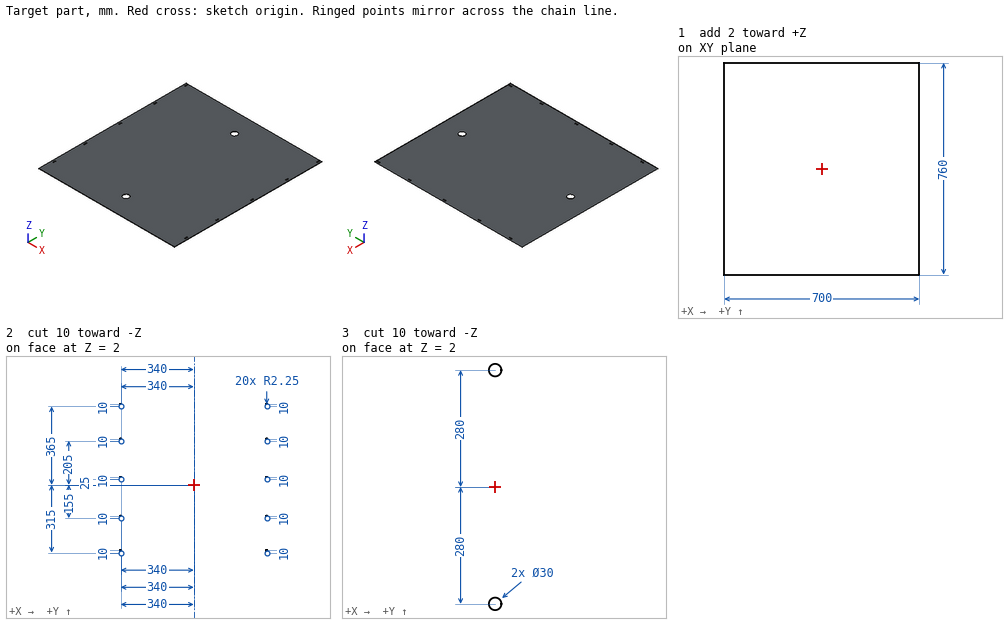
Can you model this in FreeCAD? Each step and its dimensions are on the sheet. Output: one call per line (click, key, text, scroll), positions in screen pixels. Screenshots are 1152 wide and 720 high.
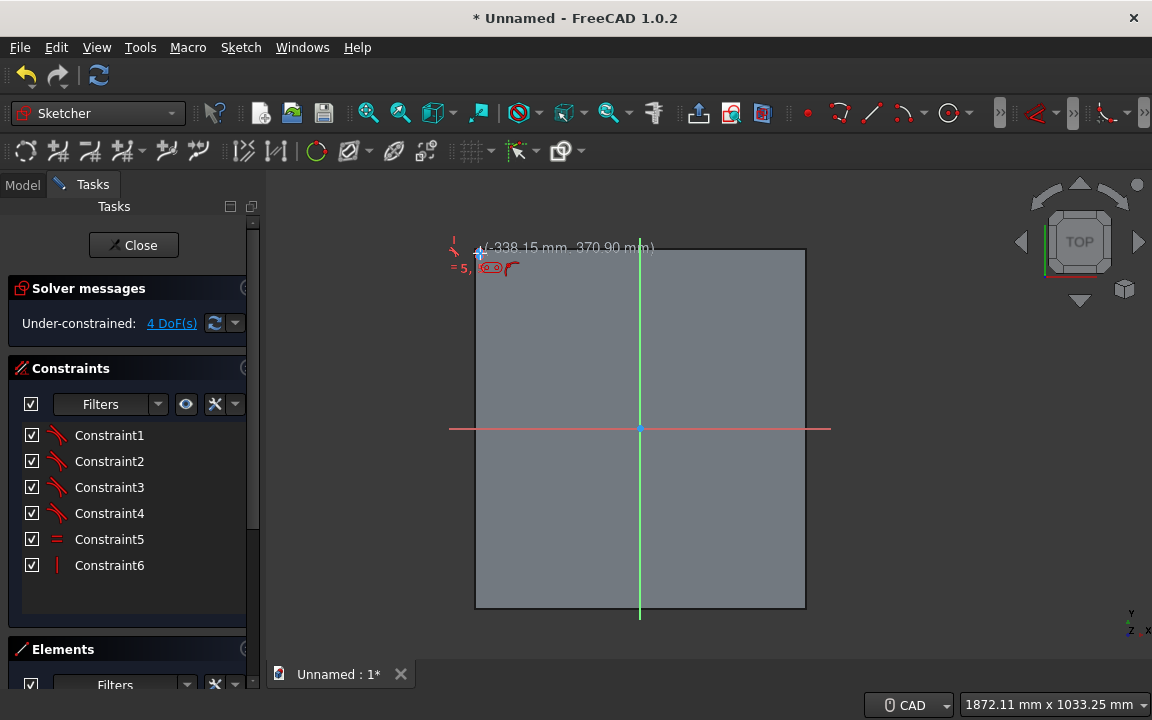
scroll(479, 332, up, 16)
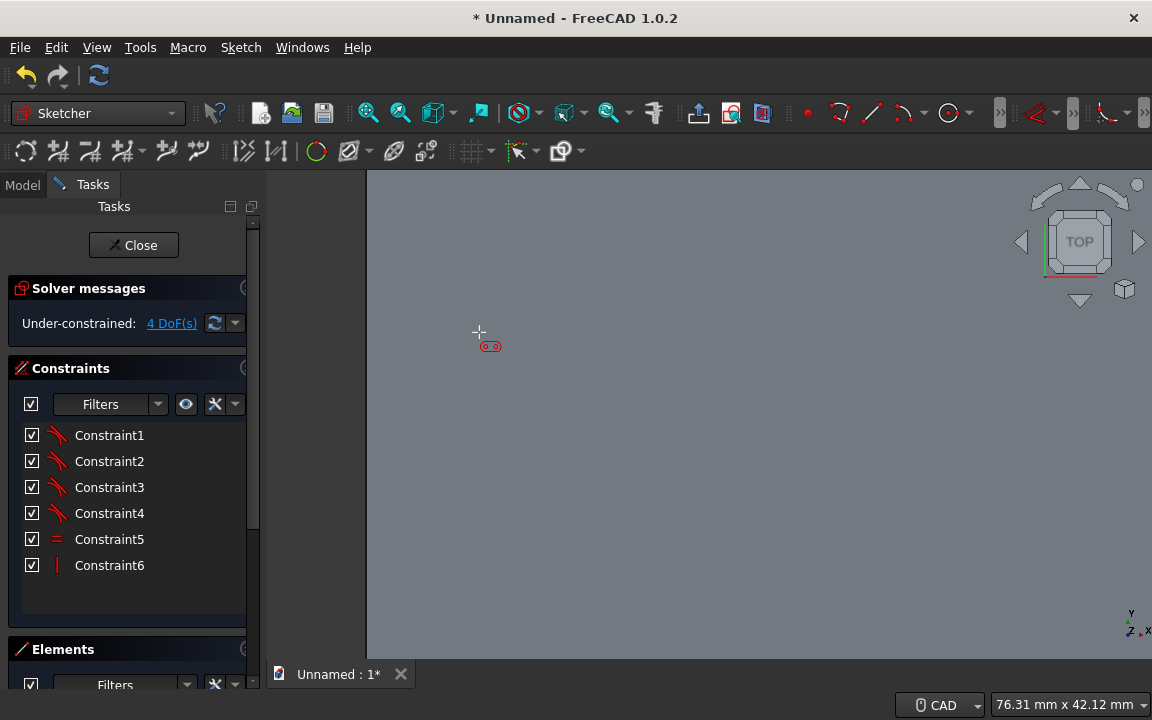
scroll(479, 332, down, 16)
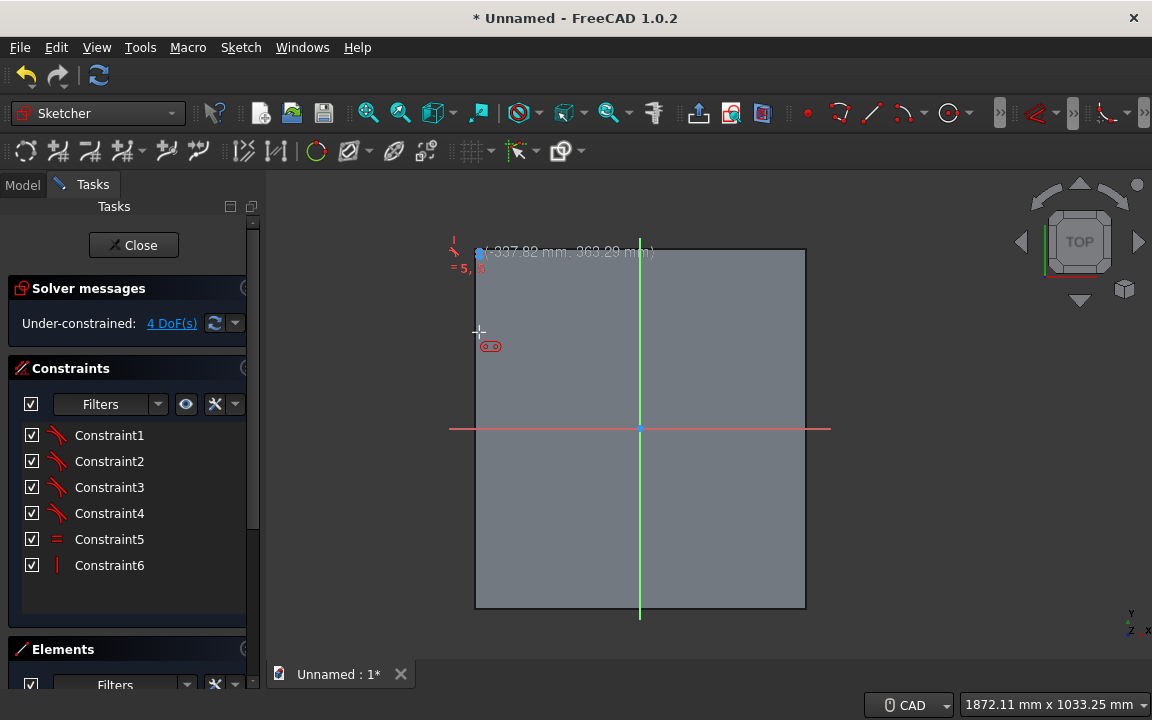
click(479, 332)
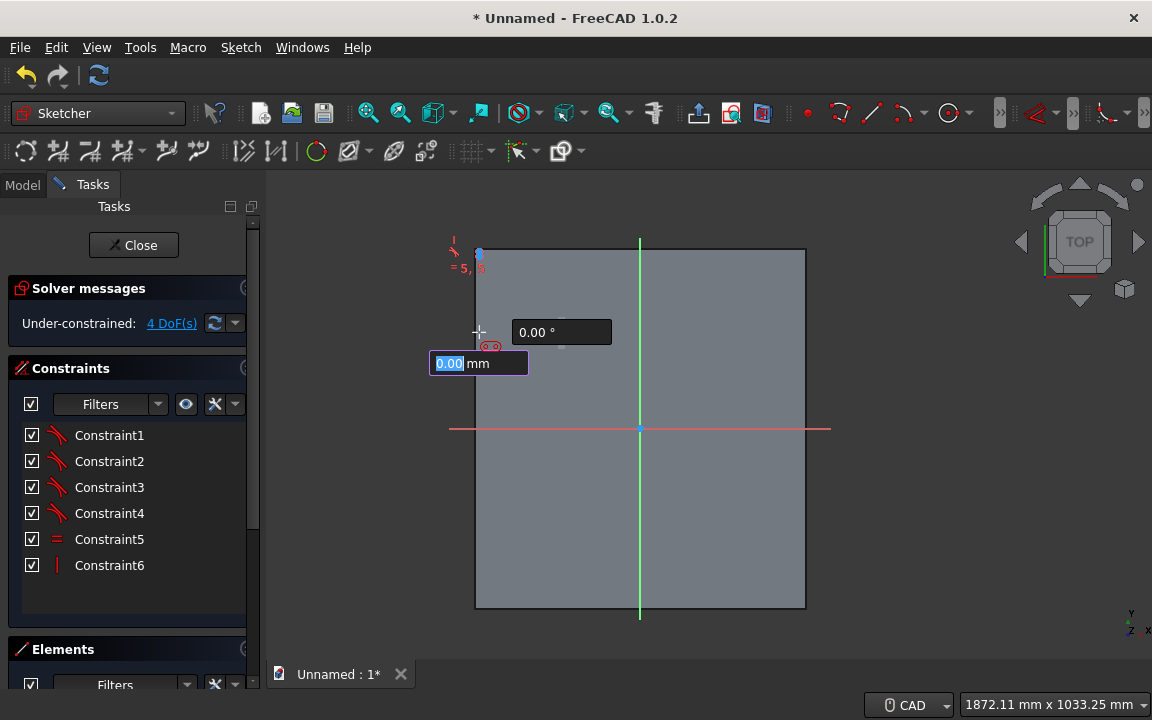
scroll(479, 327, up, 7)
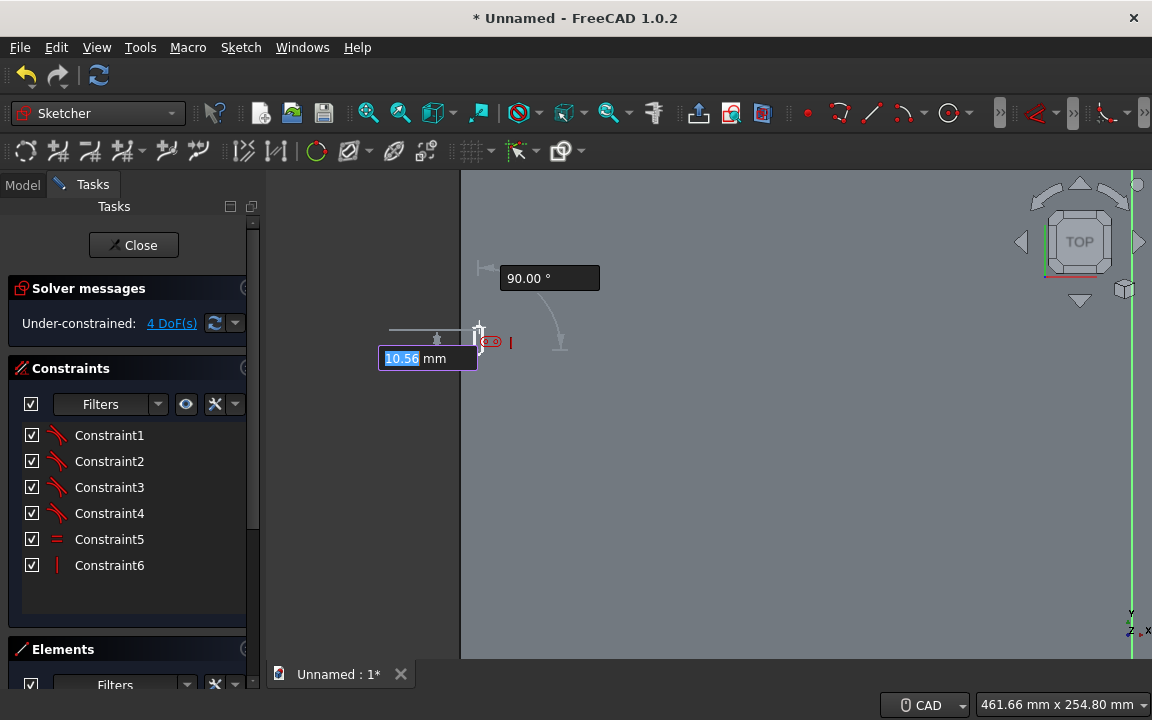
click(478, 326)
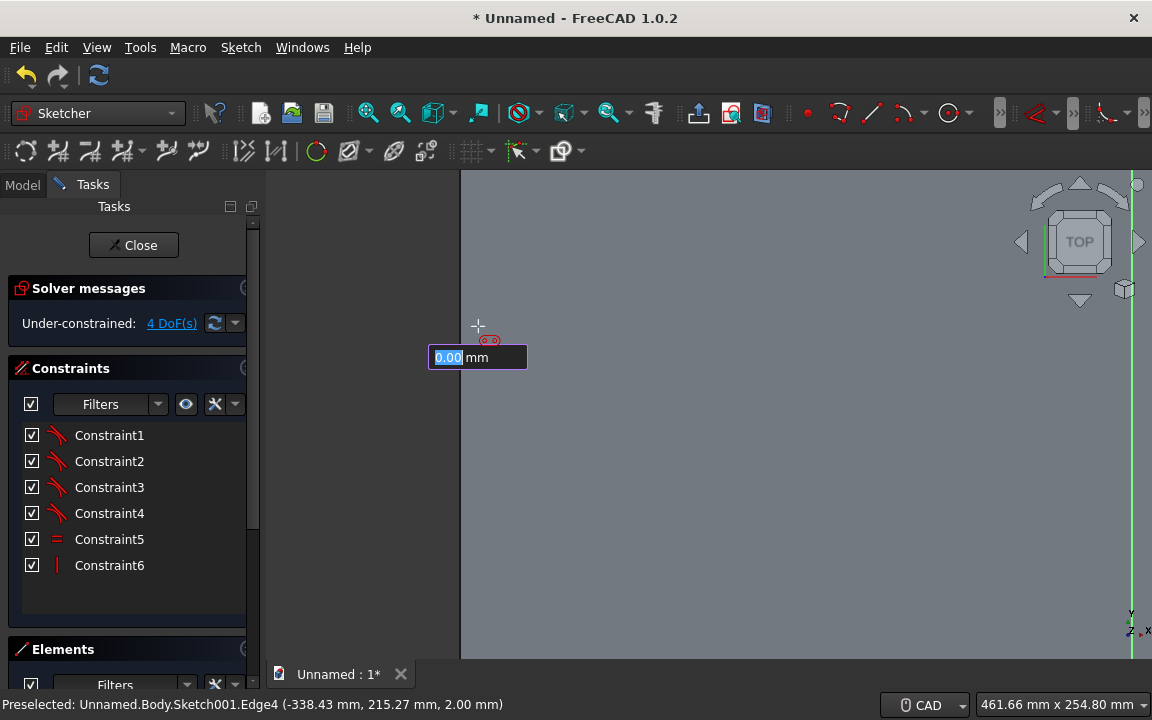
scroll(475, 336, up, 7)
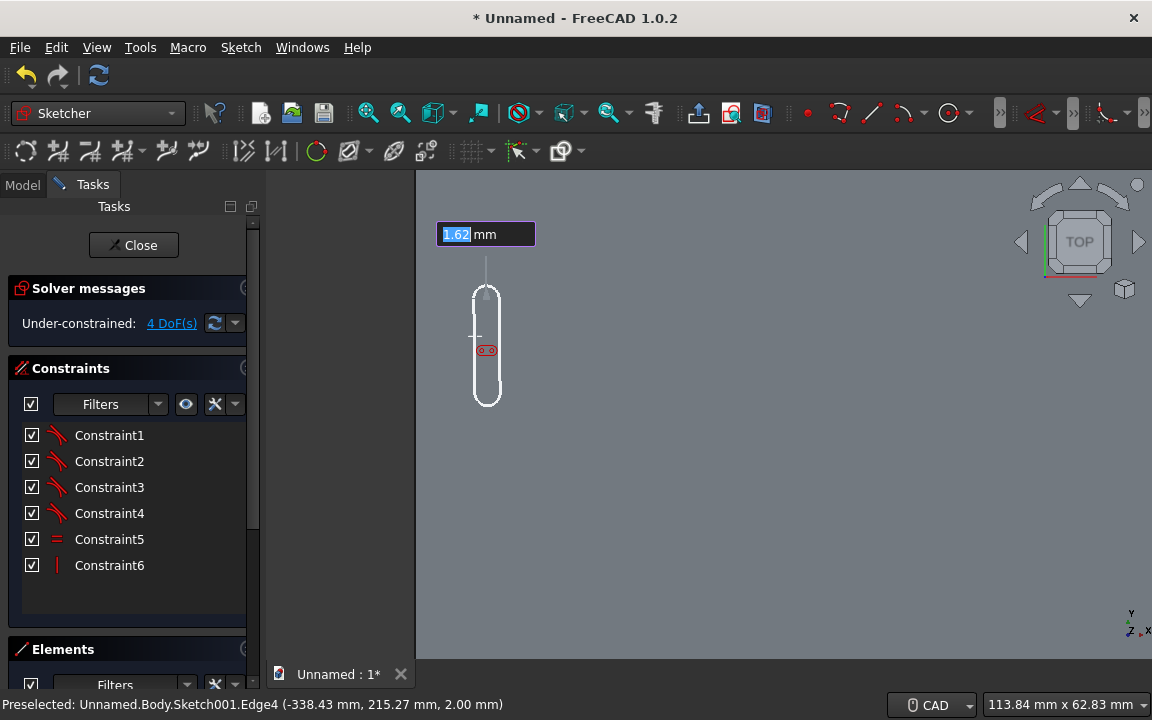
click(476, 333)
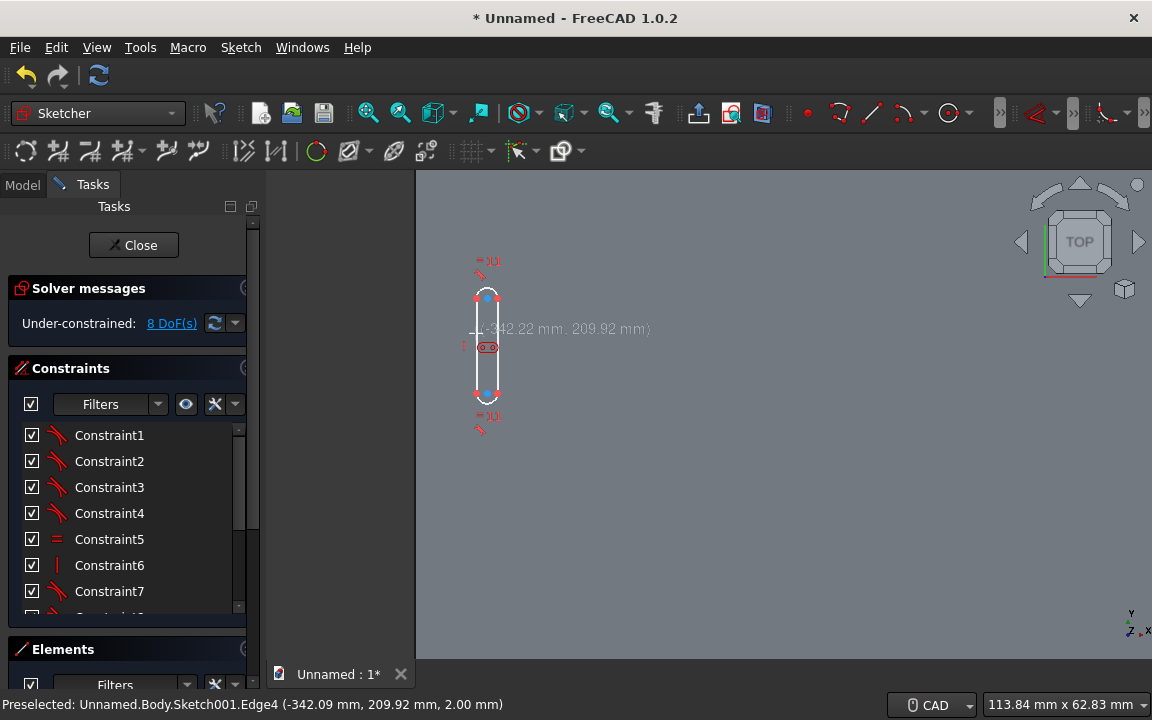
scroll(479, 329, down, 14)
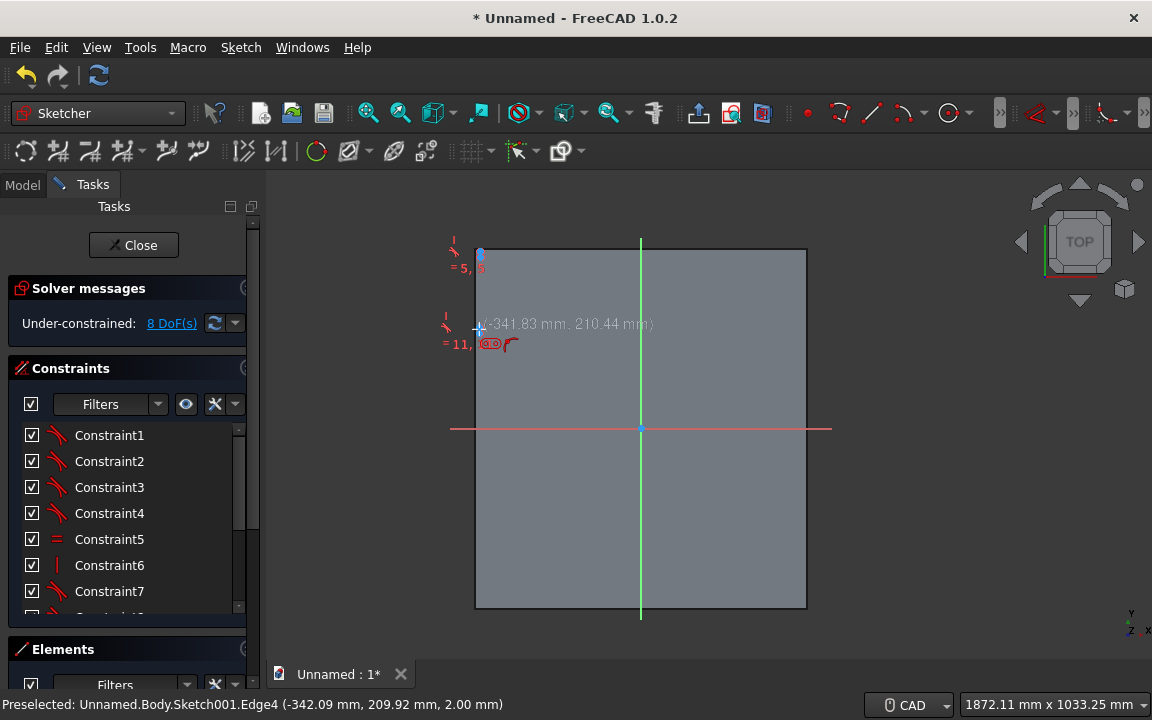
scroll(480, 417, up, 16)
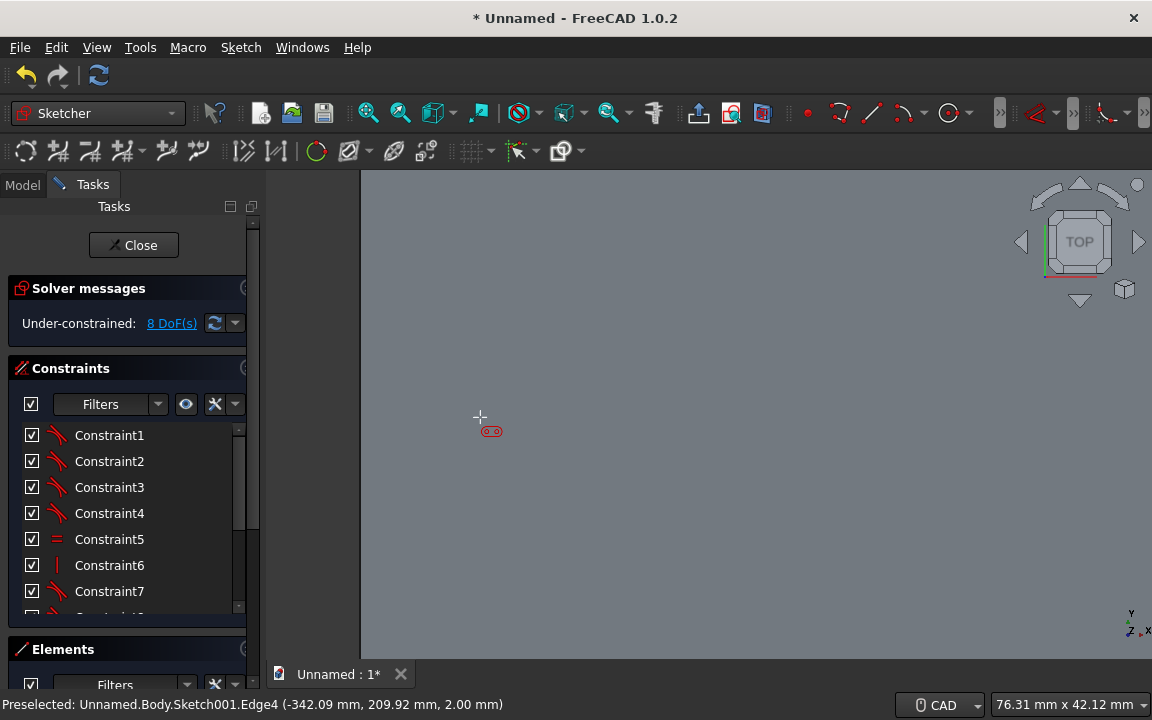
scroll(480, 417, down, 16)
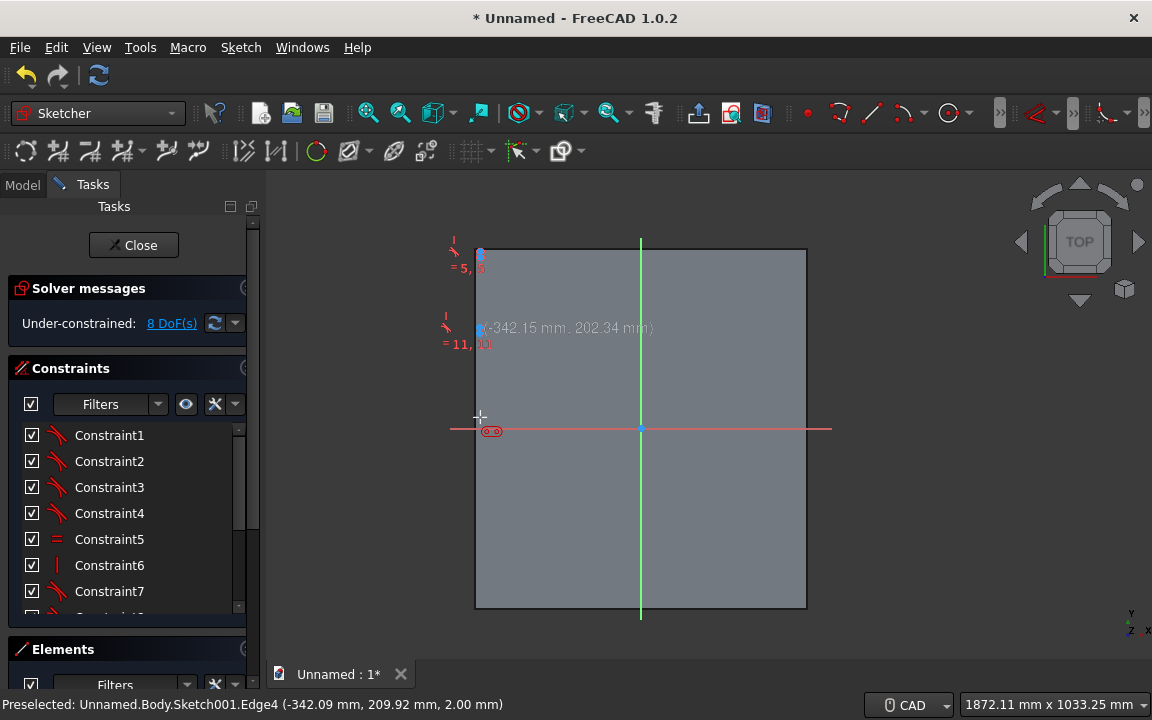
scroll(480, 417, up, 2)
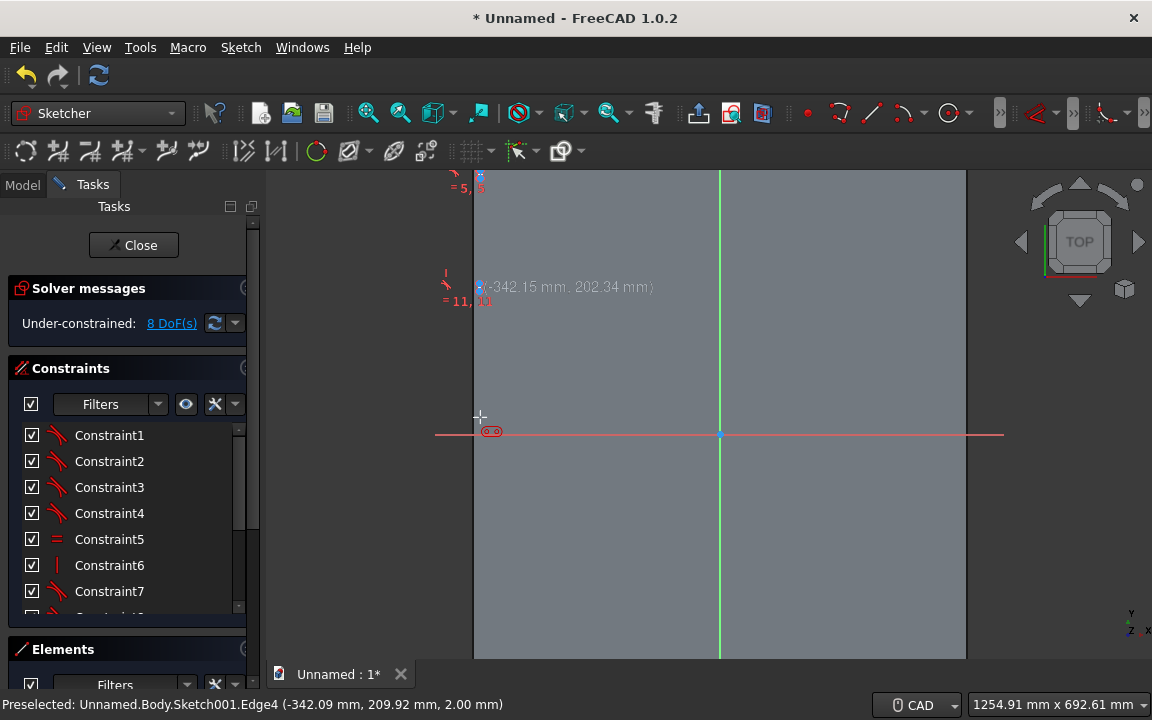
click(480, 417)